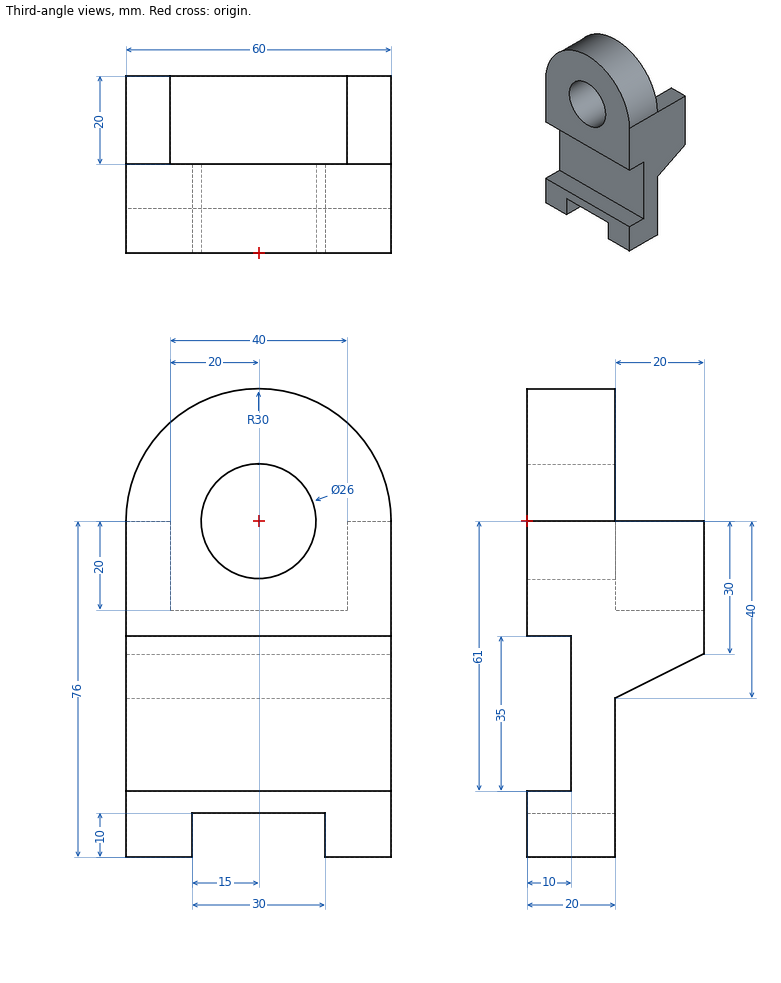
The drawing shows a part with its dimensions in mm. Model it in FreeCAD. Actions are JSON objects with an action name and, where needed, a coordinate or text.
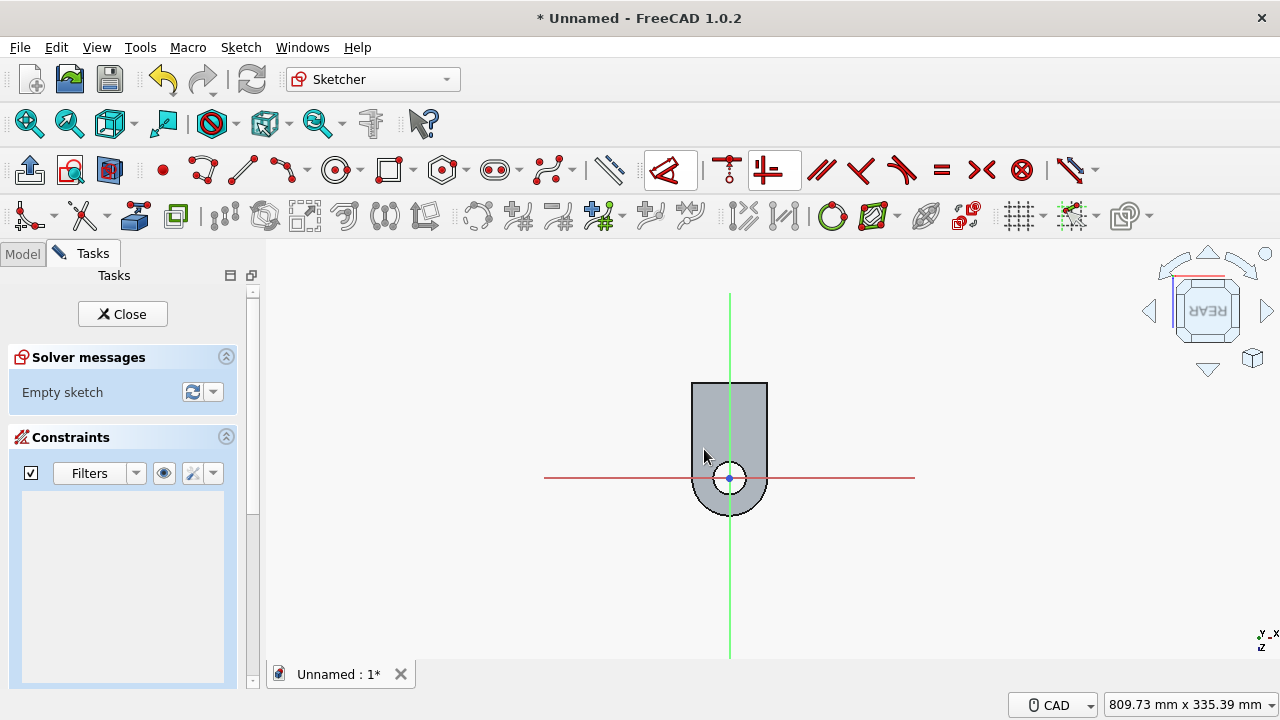
{"action": "scroll", "coordinate": [731, 385], "scroll_direction": "up", "scroll_amount": 14}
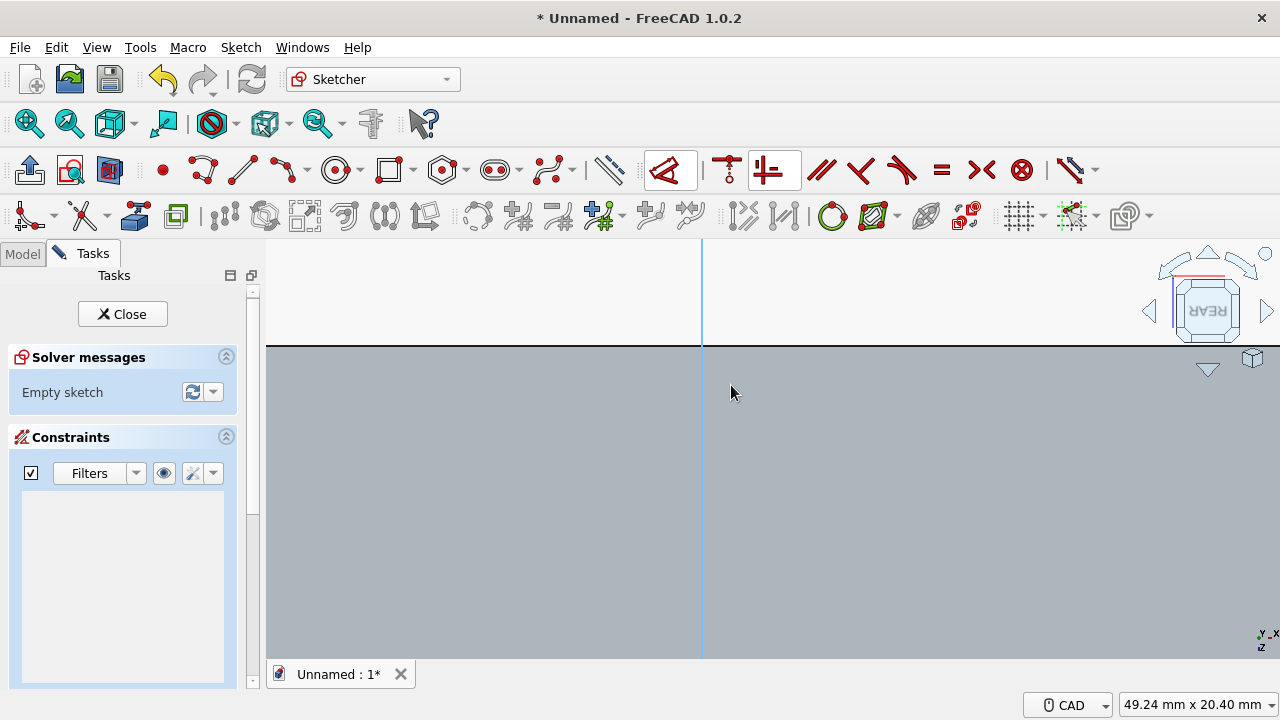
{"action": "key", "text": "g r"}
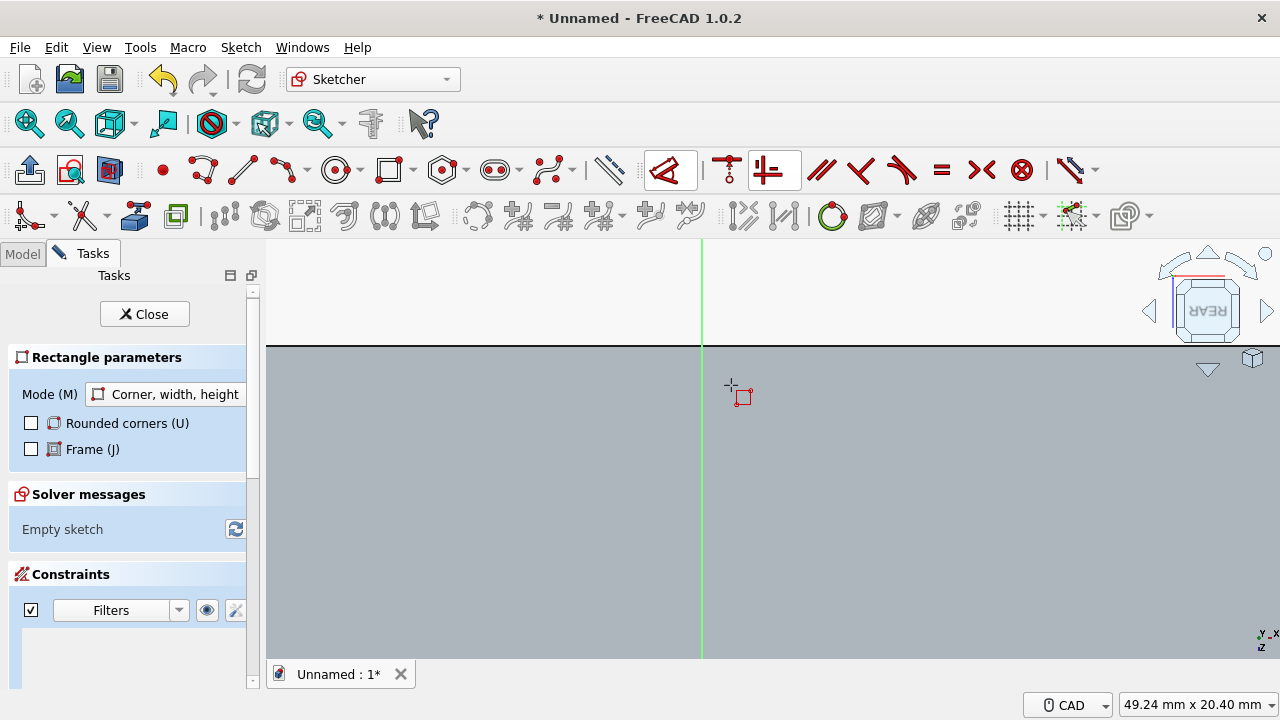
{"action": "left_click", "coordinate": [393, 346]}
{"action": "left_click", "coordinate": [1011, 552]}
{"action": "key", "text": "Escape"}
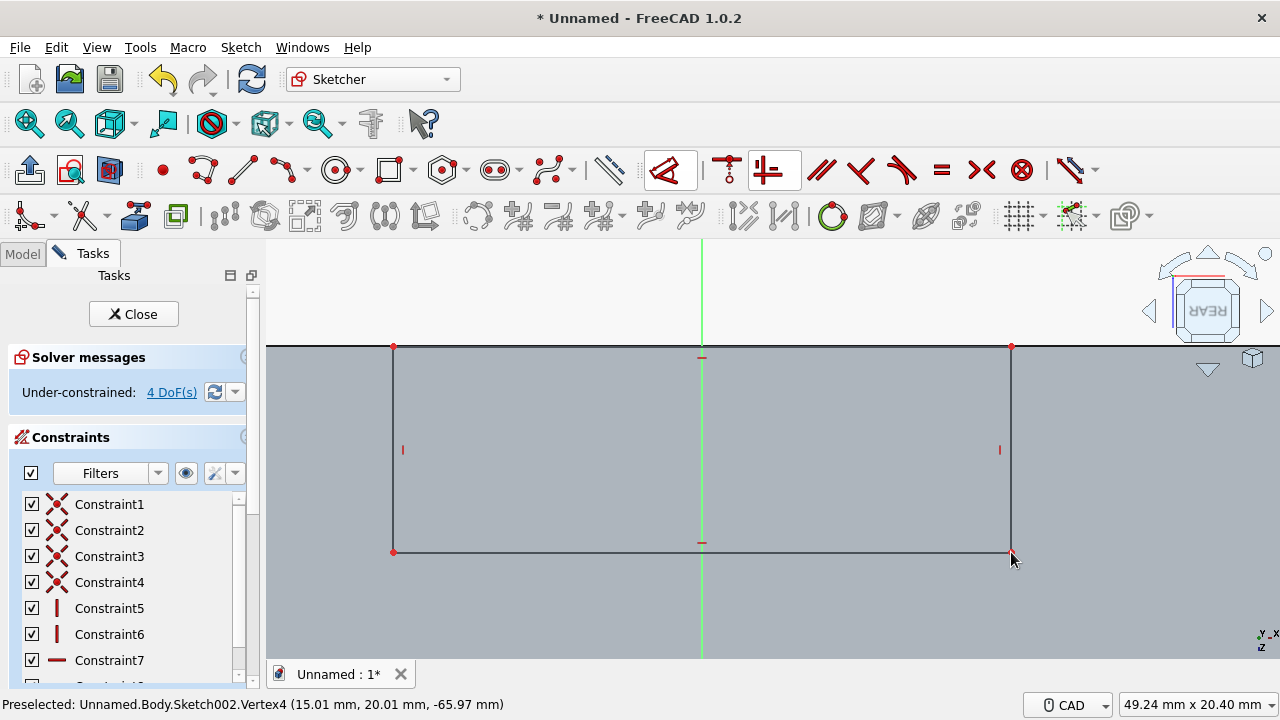
{"action": "left_click", "coordinate": [393, 409]}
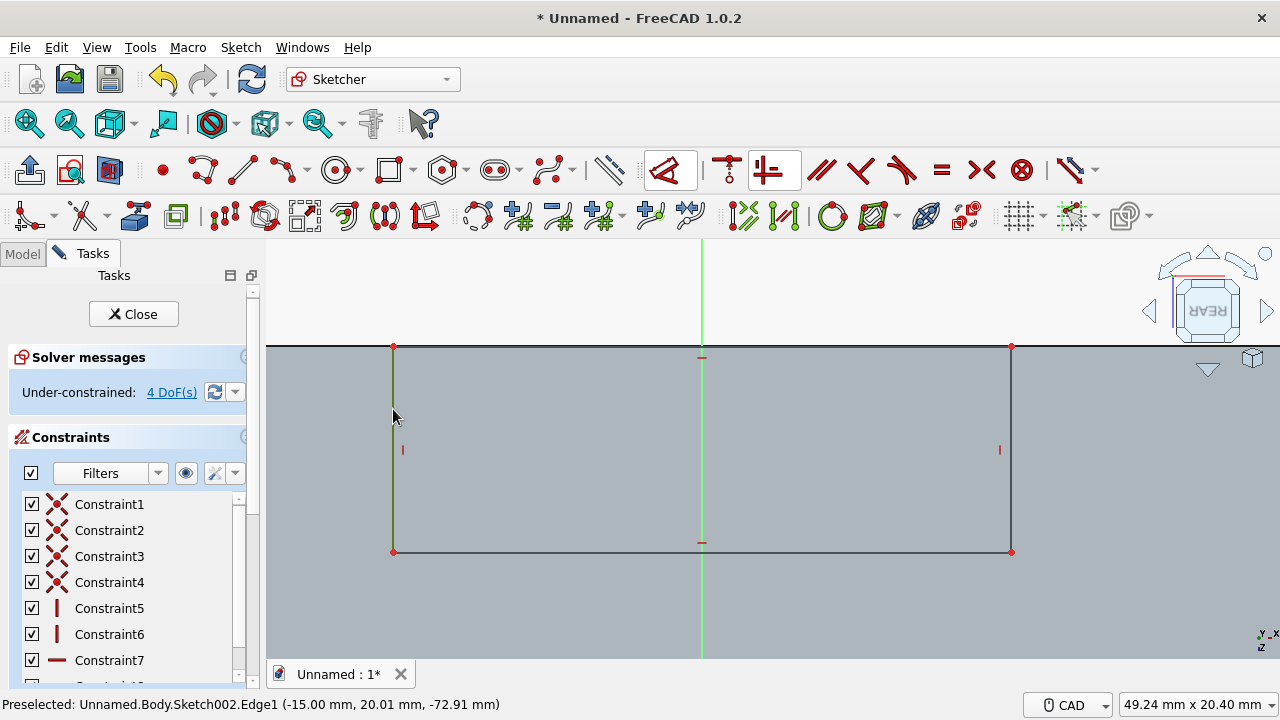
{"action": "key", "text": "i"}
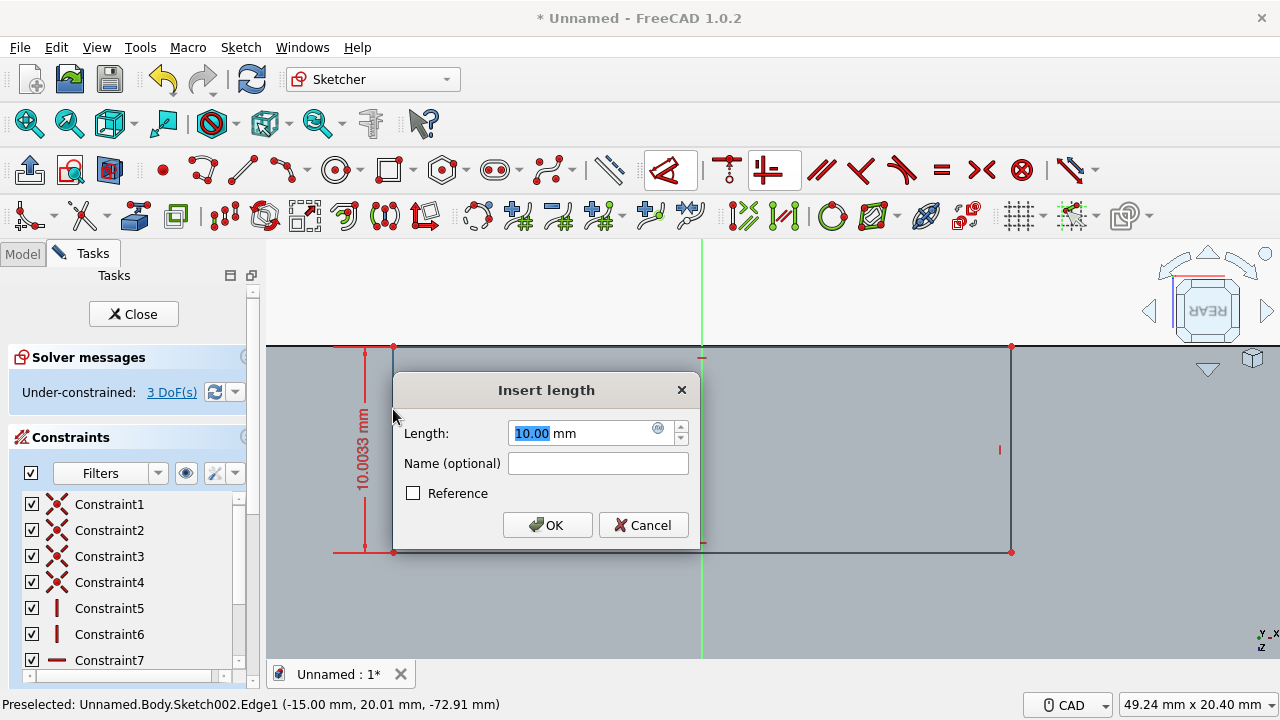
{"action": "type", "text": "10"}
{"action": "key", "text": "Return"}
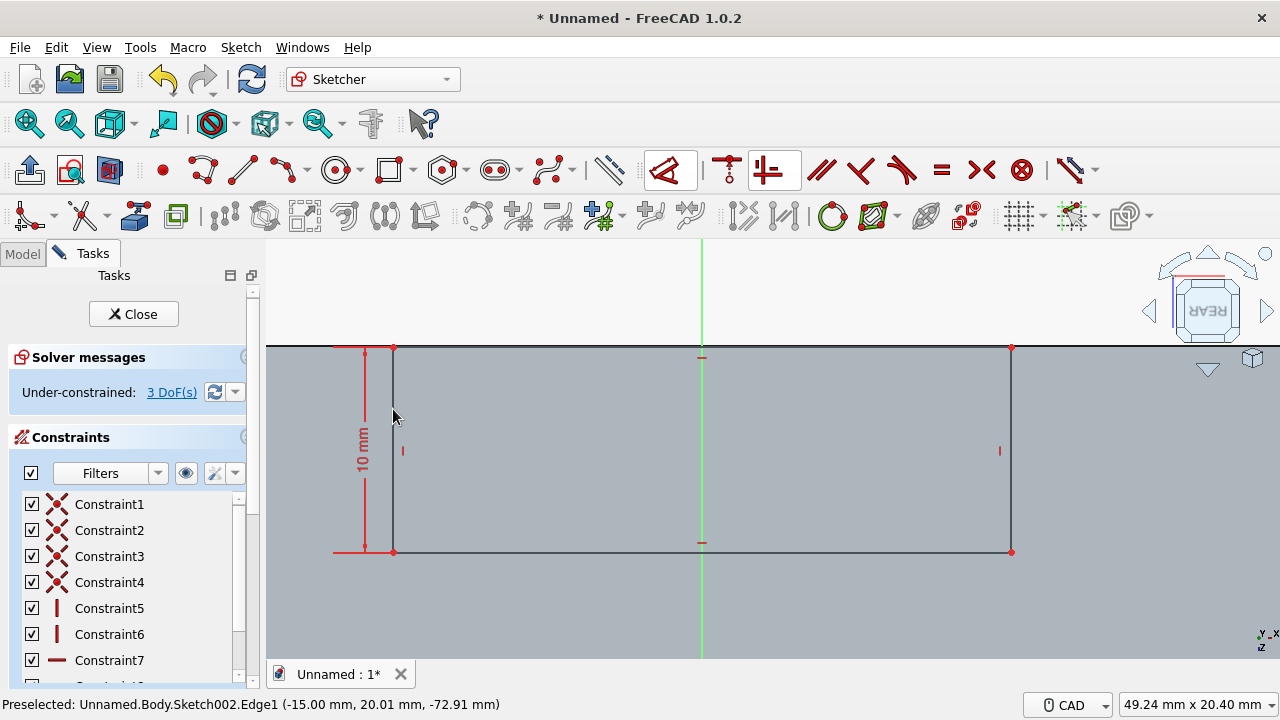
{"action": "left_click", "coordinate": [578, 553]}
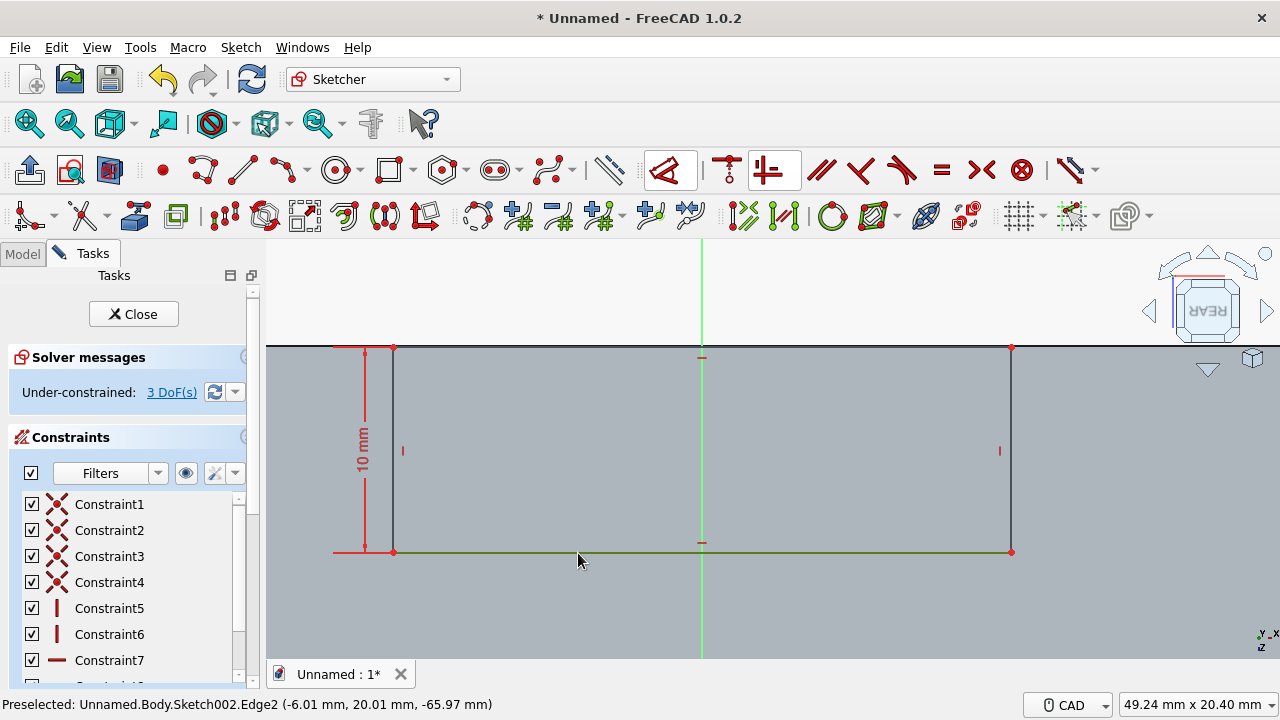
{"action": "key", "text": "l"}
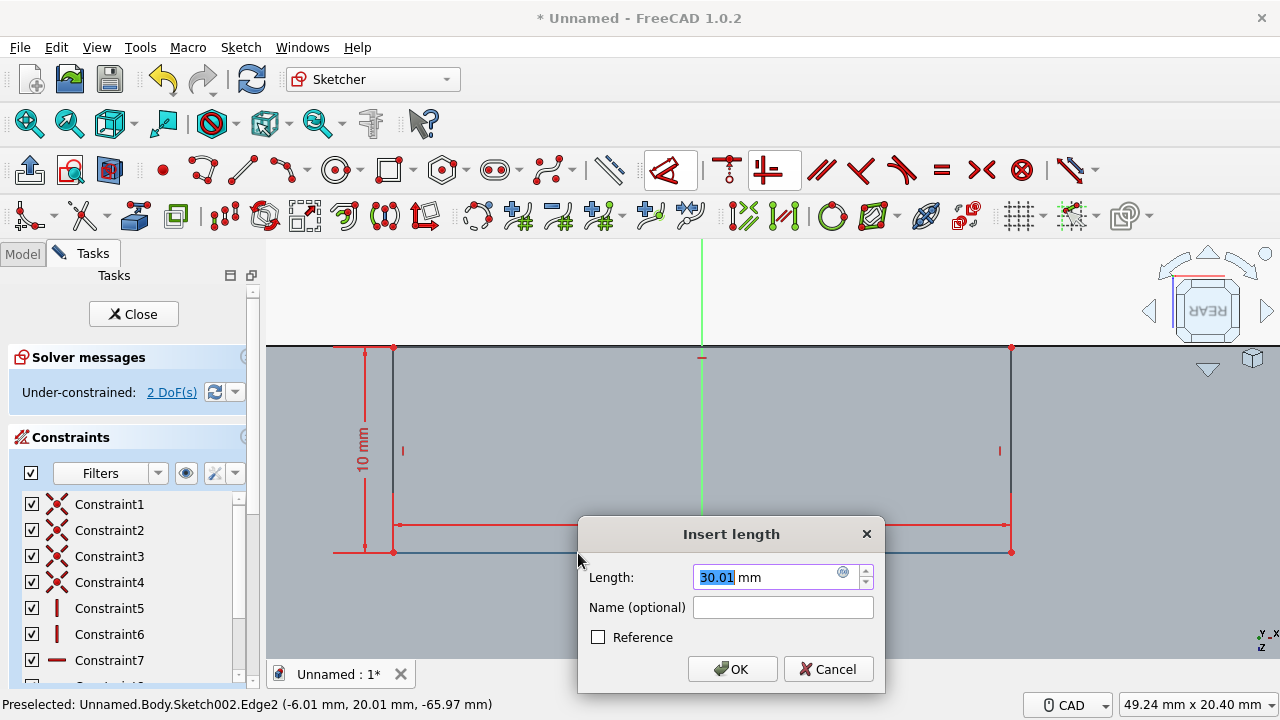
{"action": "type", "text": "30"}
{"action": "key", "text": "Return"}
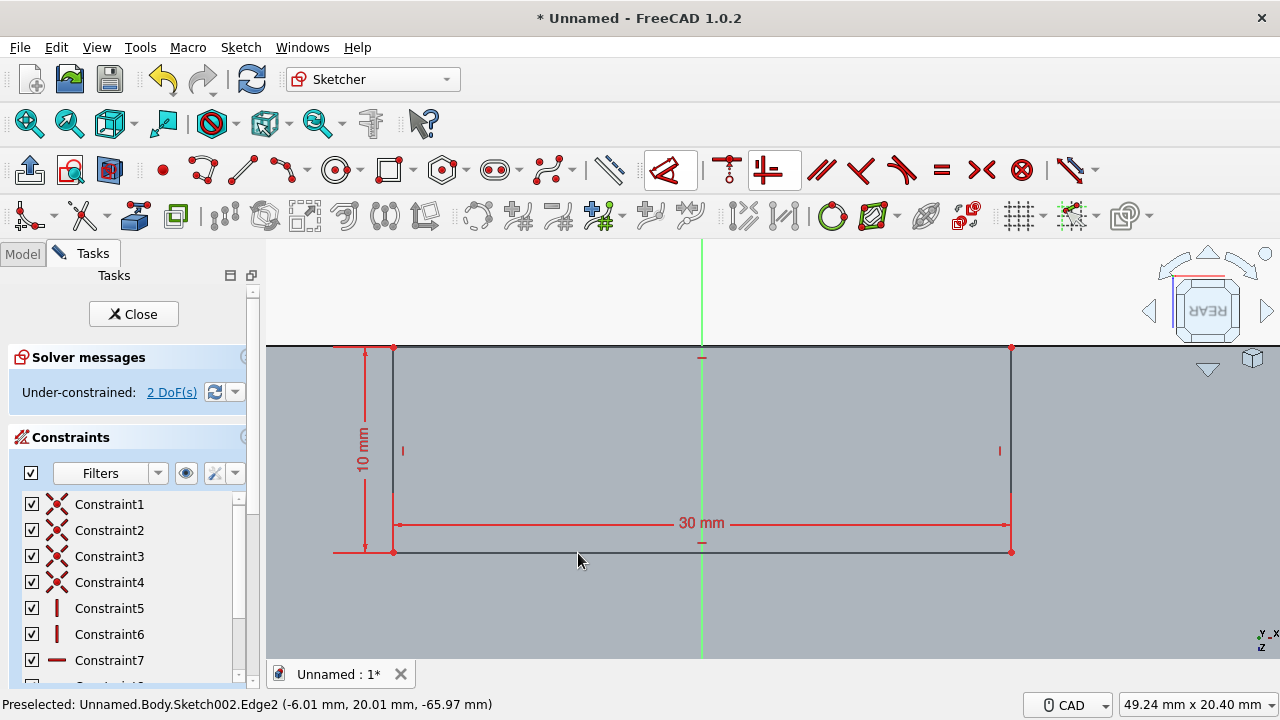
{"action": "left_click", "coordinate": [393, 347]}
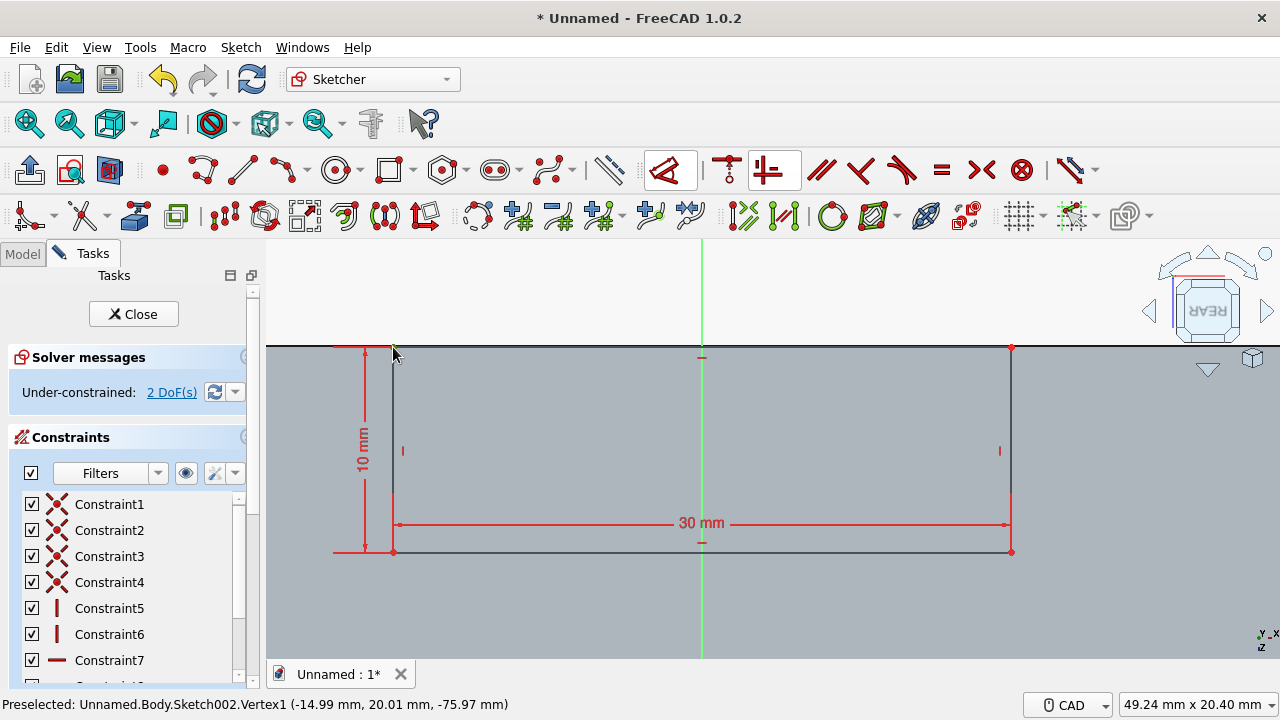
{"action": "key", "text": "l"}